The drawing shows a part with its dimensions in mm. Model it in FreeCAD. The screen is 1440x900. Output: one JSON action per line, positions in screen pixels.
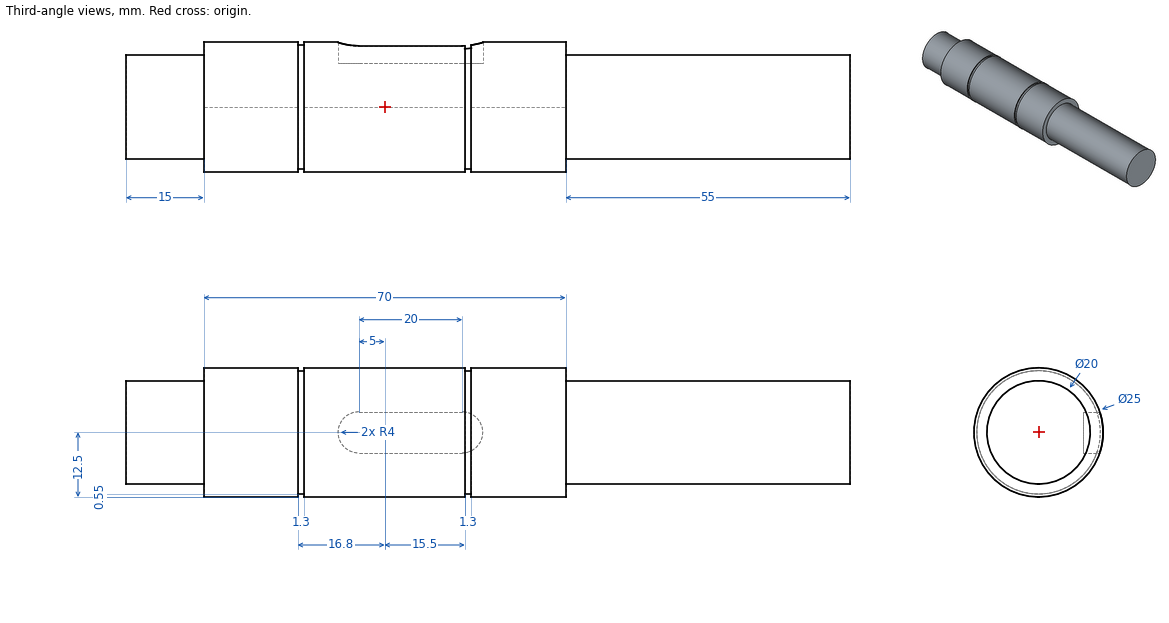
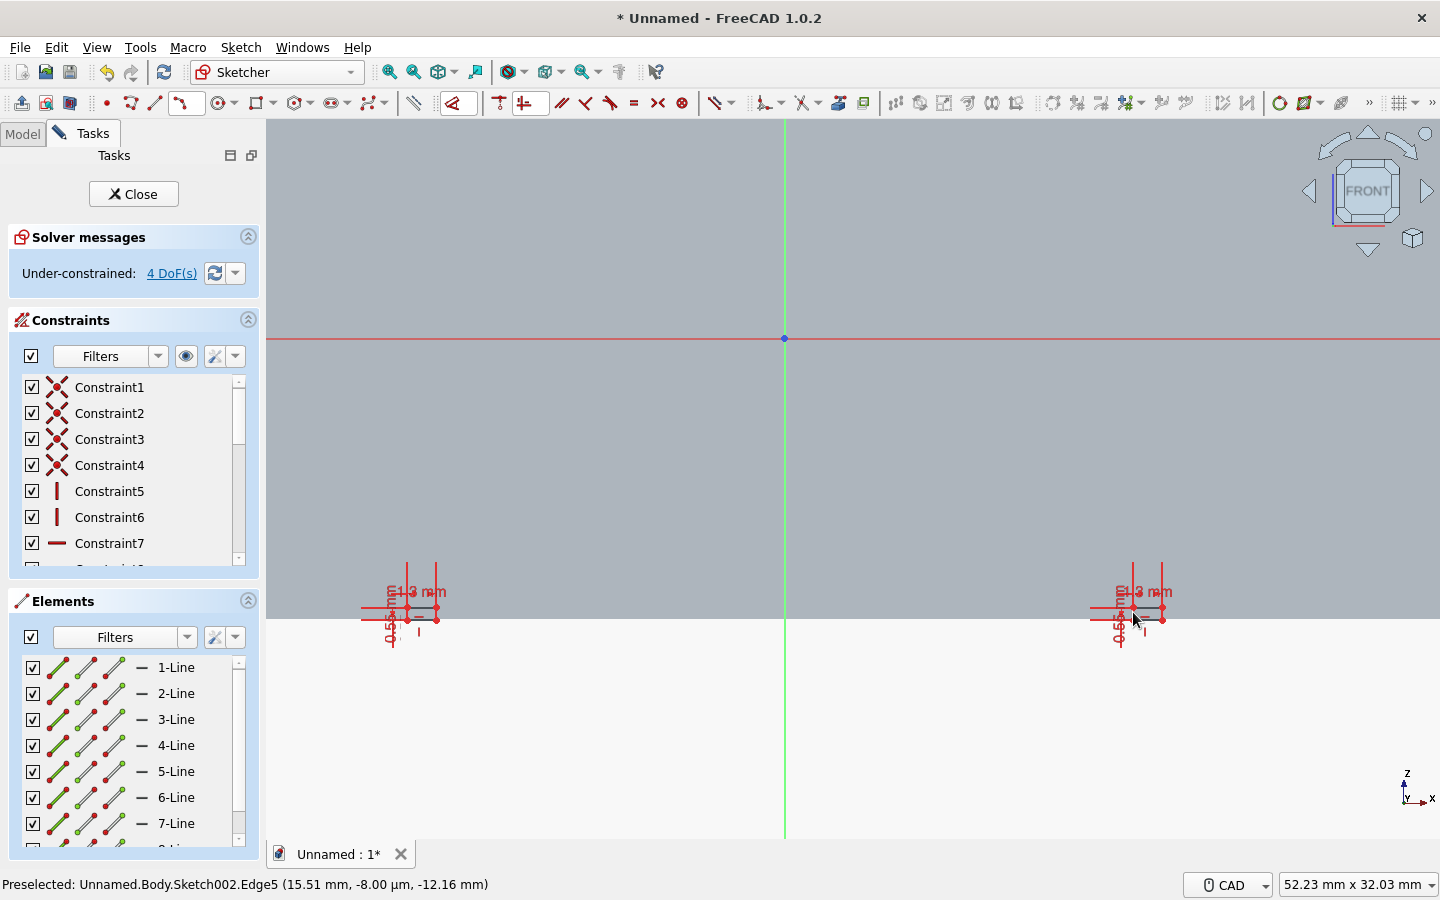
{"action": "left_click", "coordinate": [407, 608]}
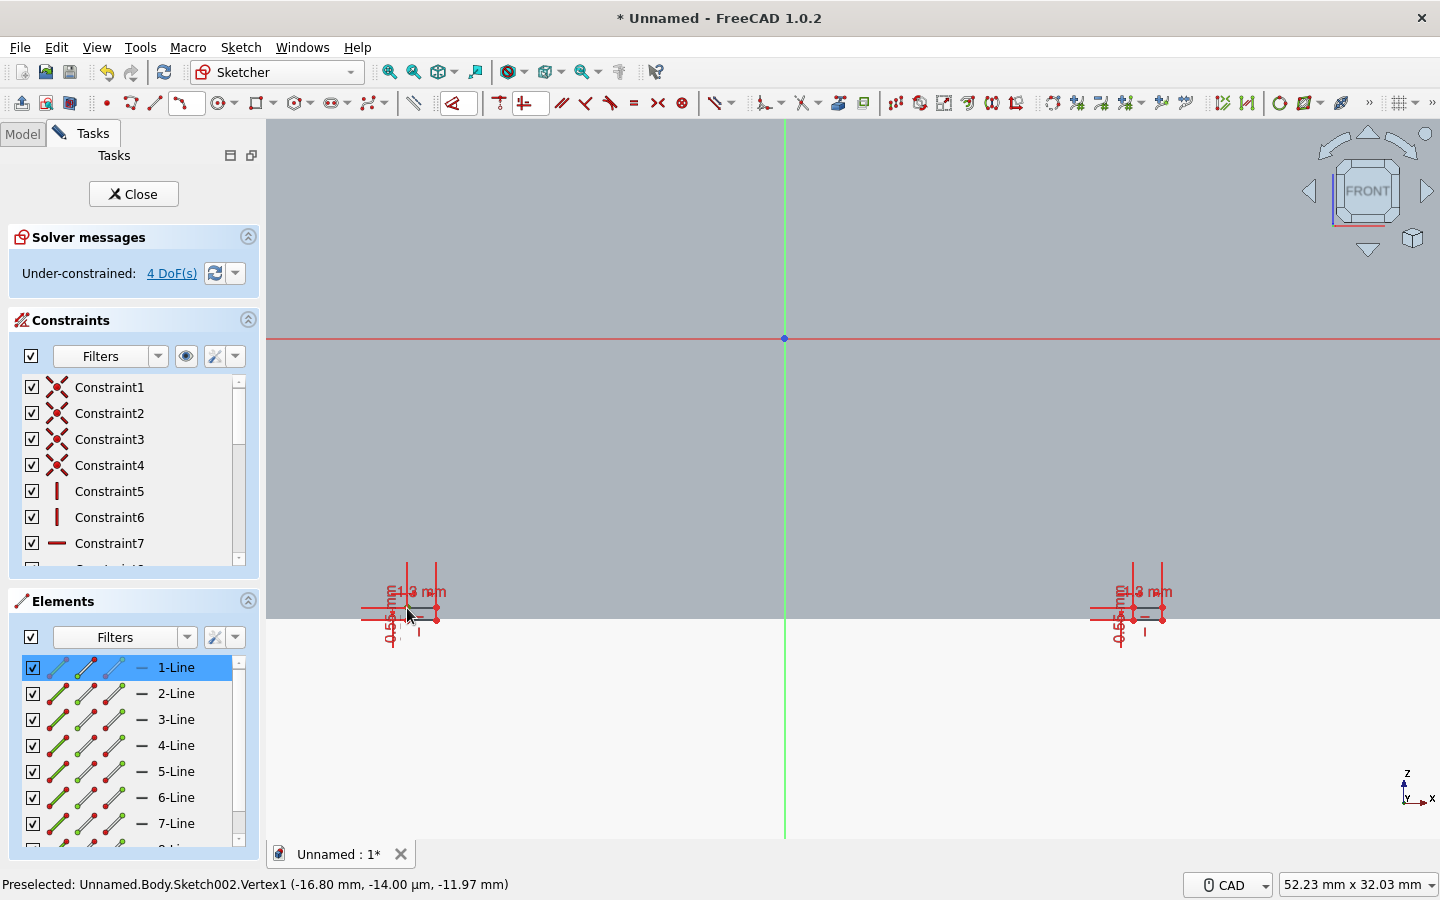
{"action": "left_click", "coordinate": [472, 104]}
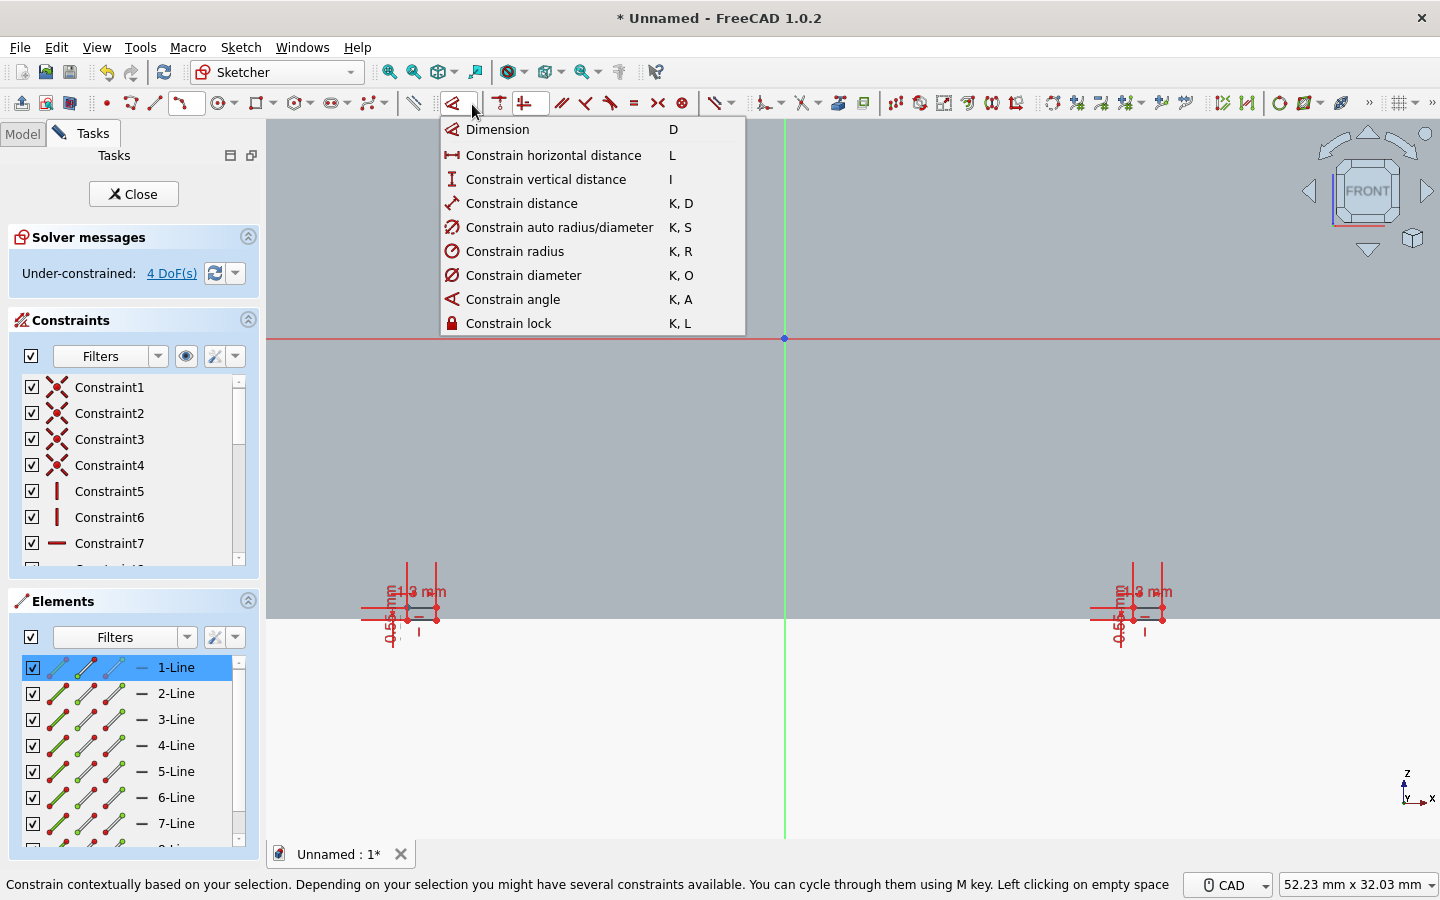
{"action": "left_click", "coordinate": [593, 155]}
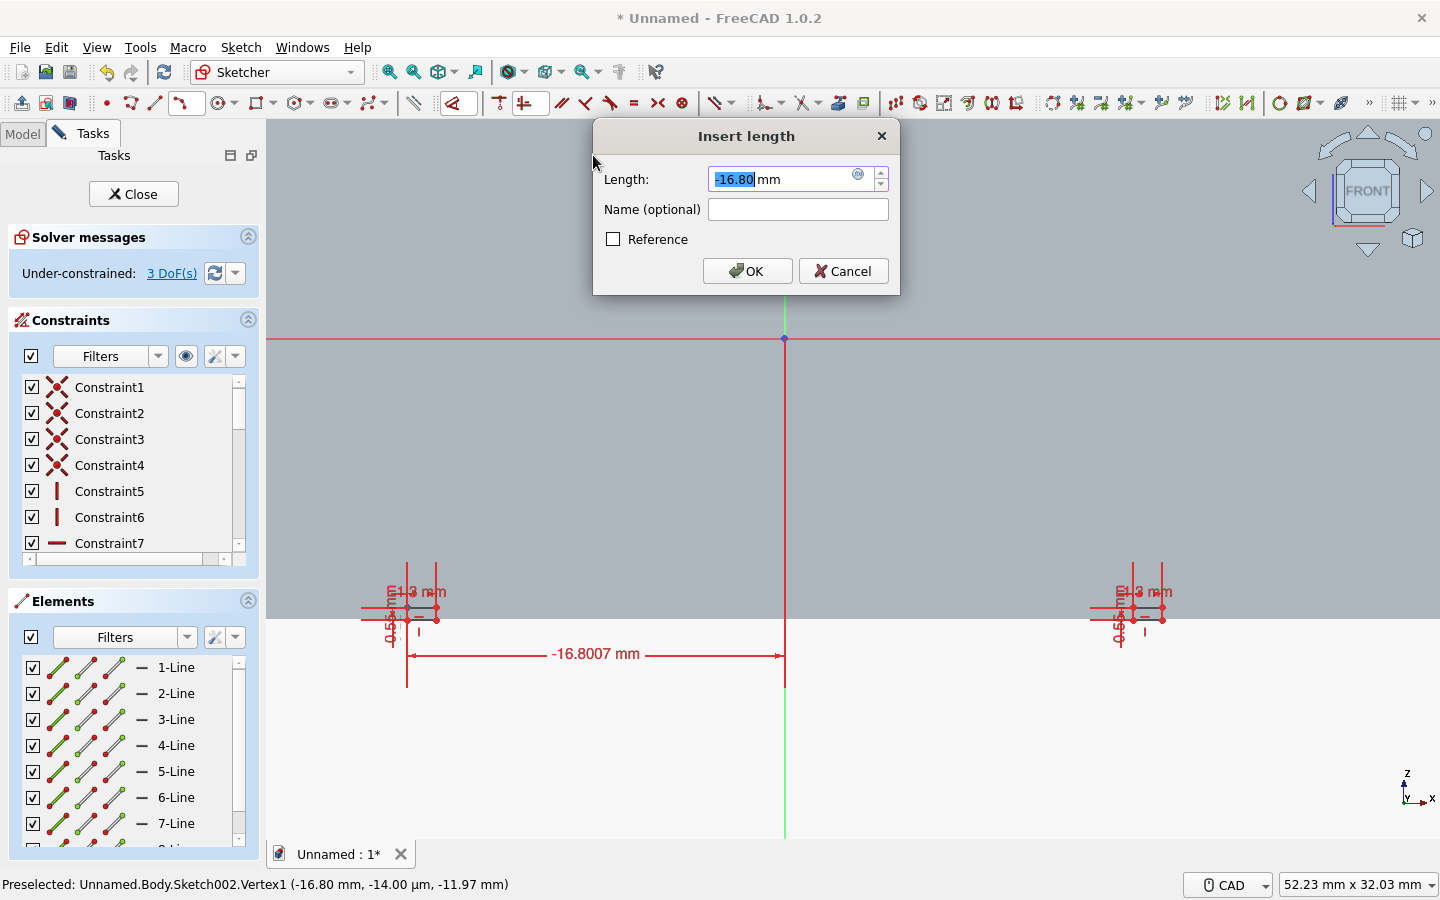
{"action": "type", "text": "-16.8"}
{"action": "key", "text": "Return"}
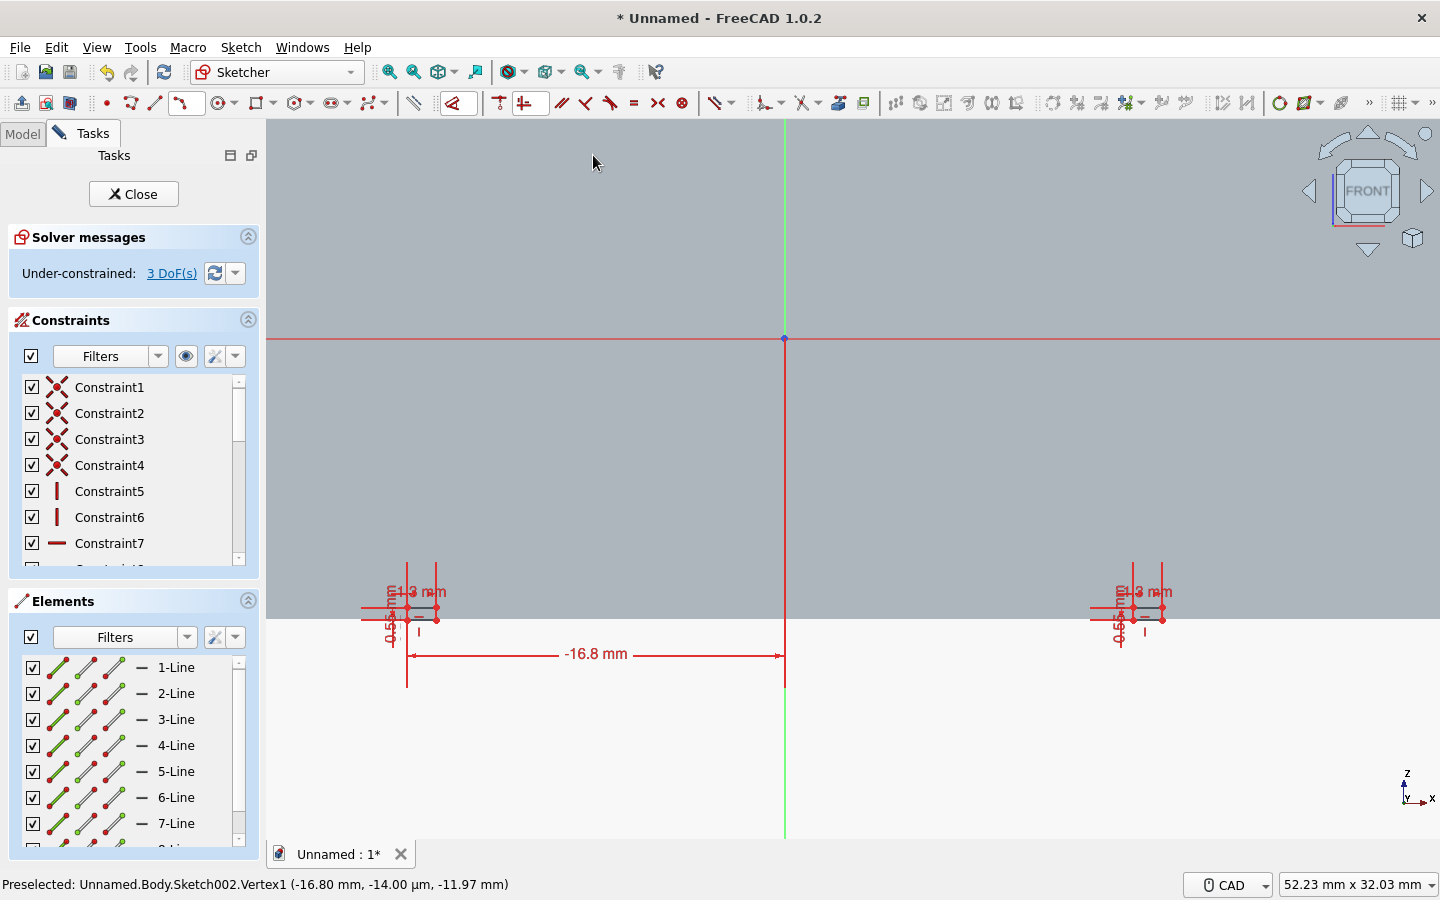
{"action": "left_click", "coordinate": [407, 620]}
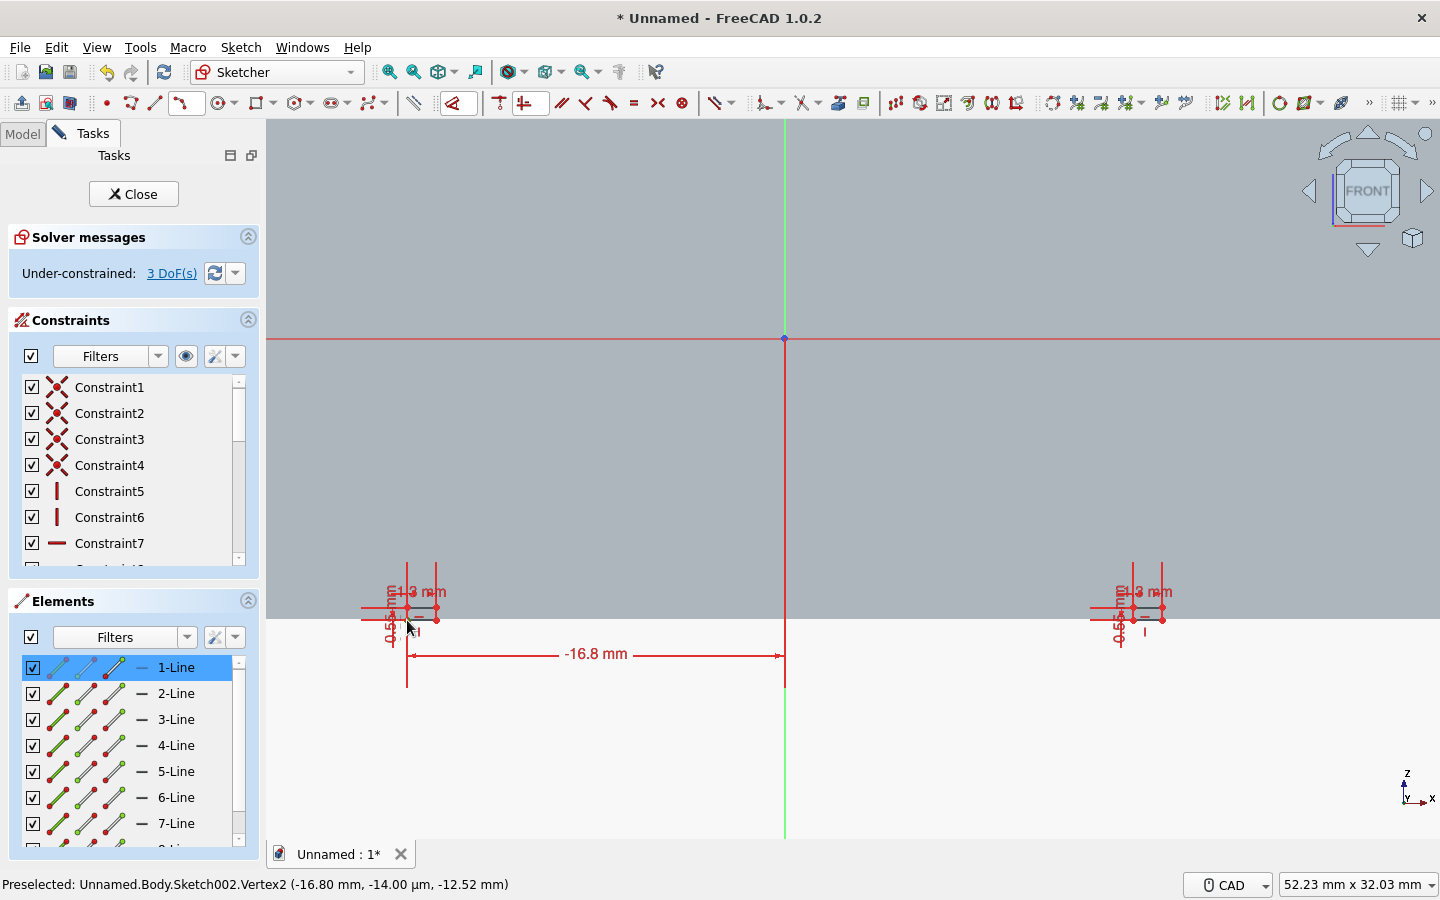
{"action": "left_click", "coordinate": [472, 104]}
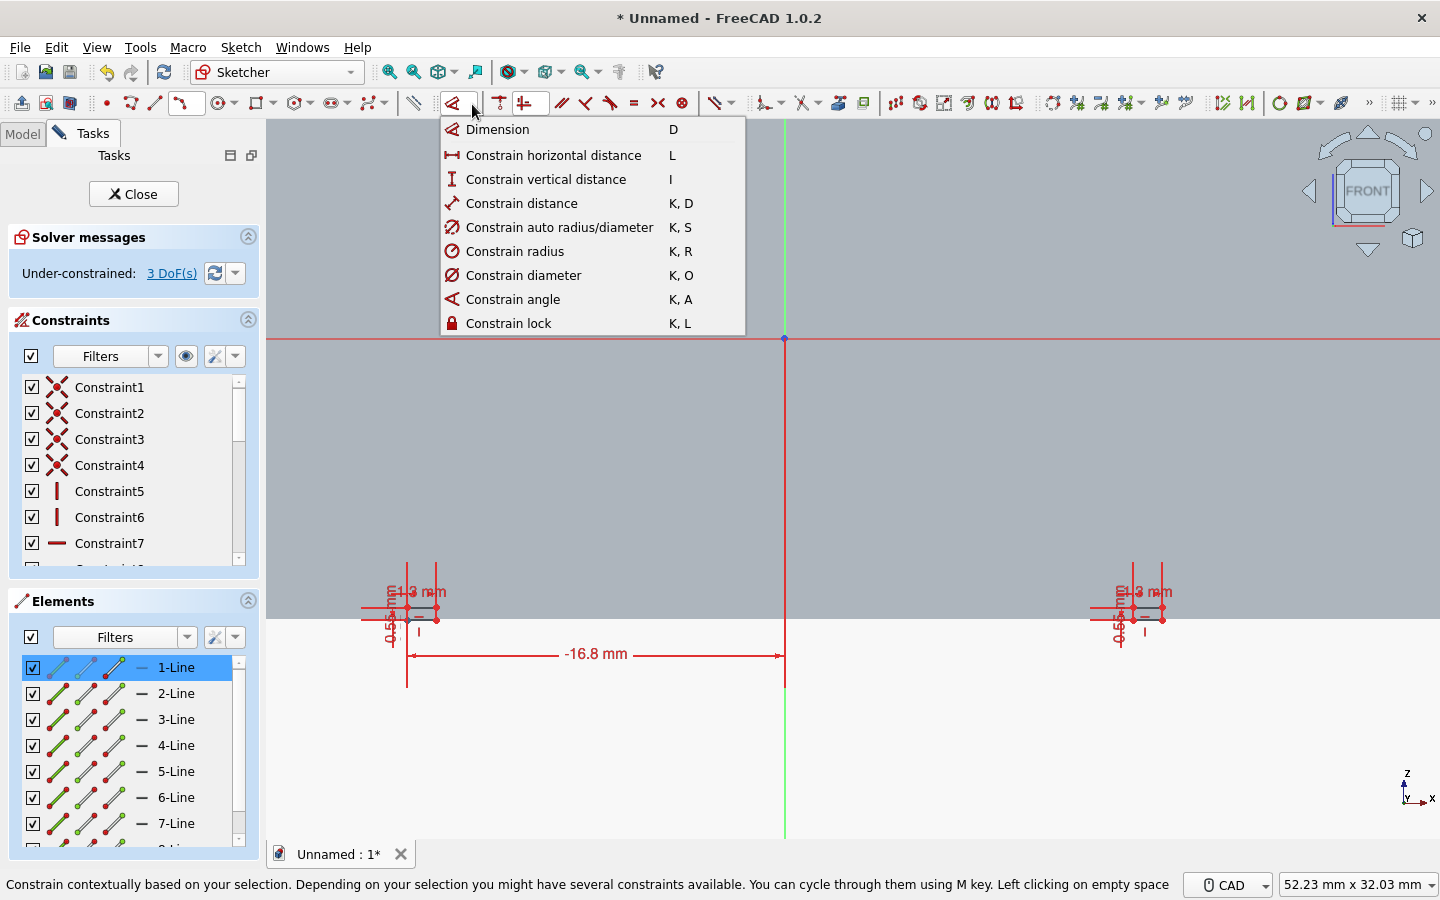
{"action": "left_click", "coordinate": [593, 179]}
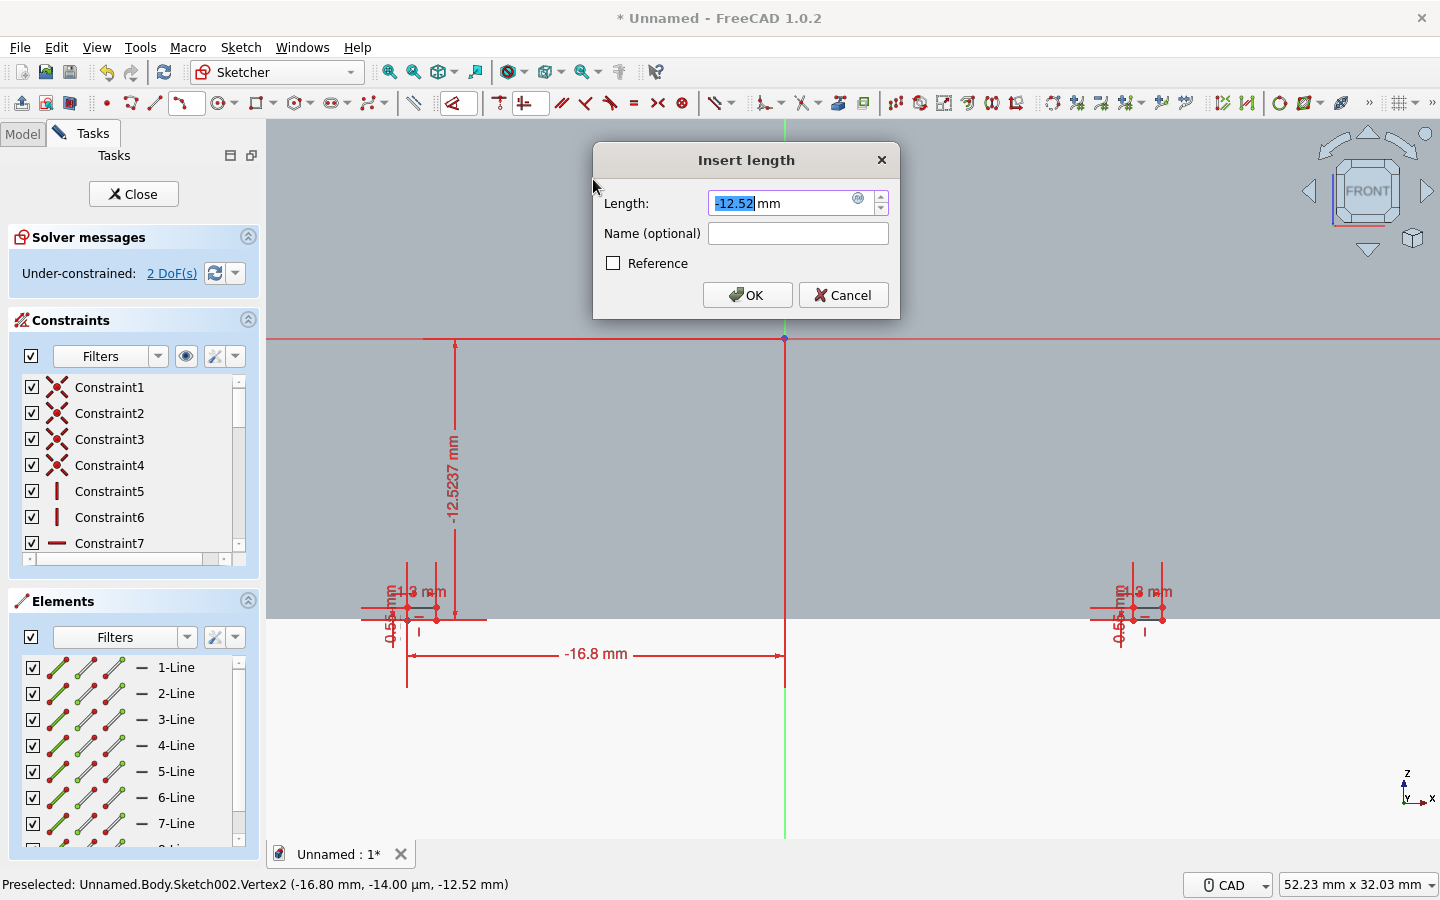
{"action": "type", "text": "-12.5"}
{"action": "key", "text": "Return"}